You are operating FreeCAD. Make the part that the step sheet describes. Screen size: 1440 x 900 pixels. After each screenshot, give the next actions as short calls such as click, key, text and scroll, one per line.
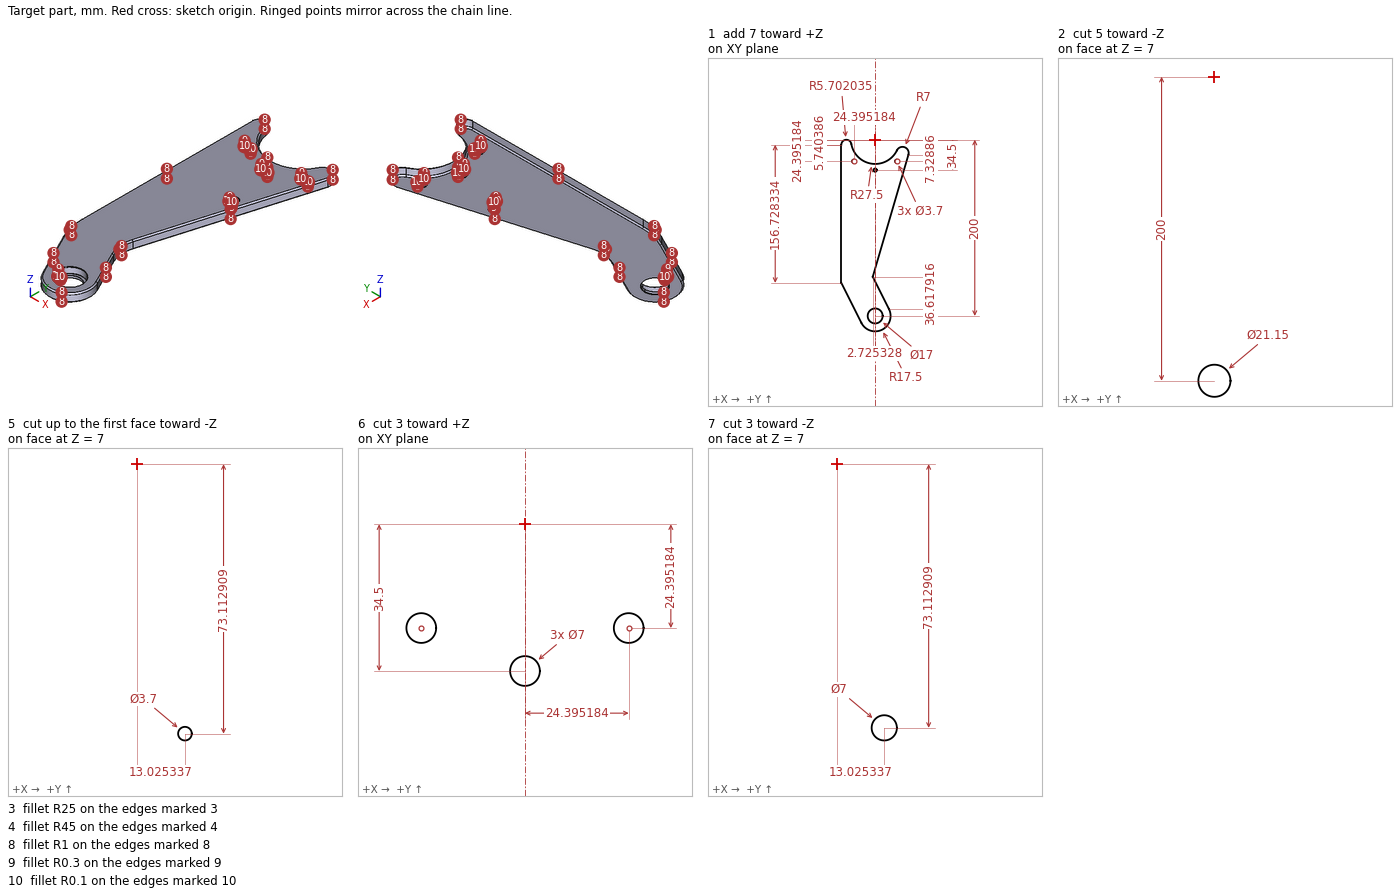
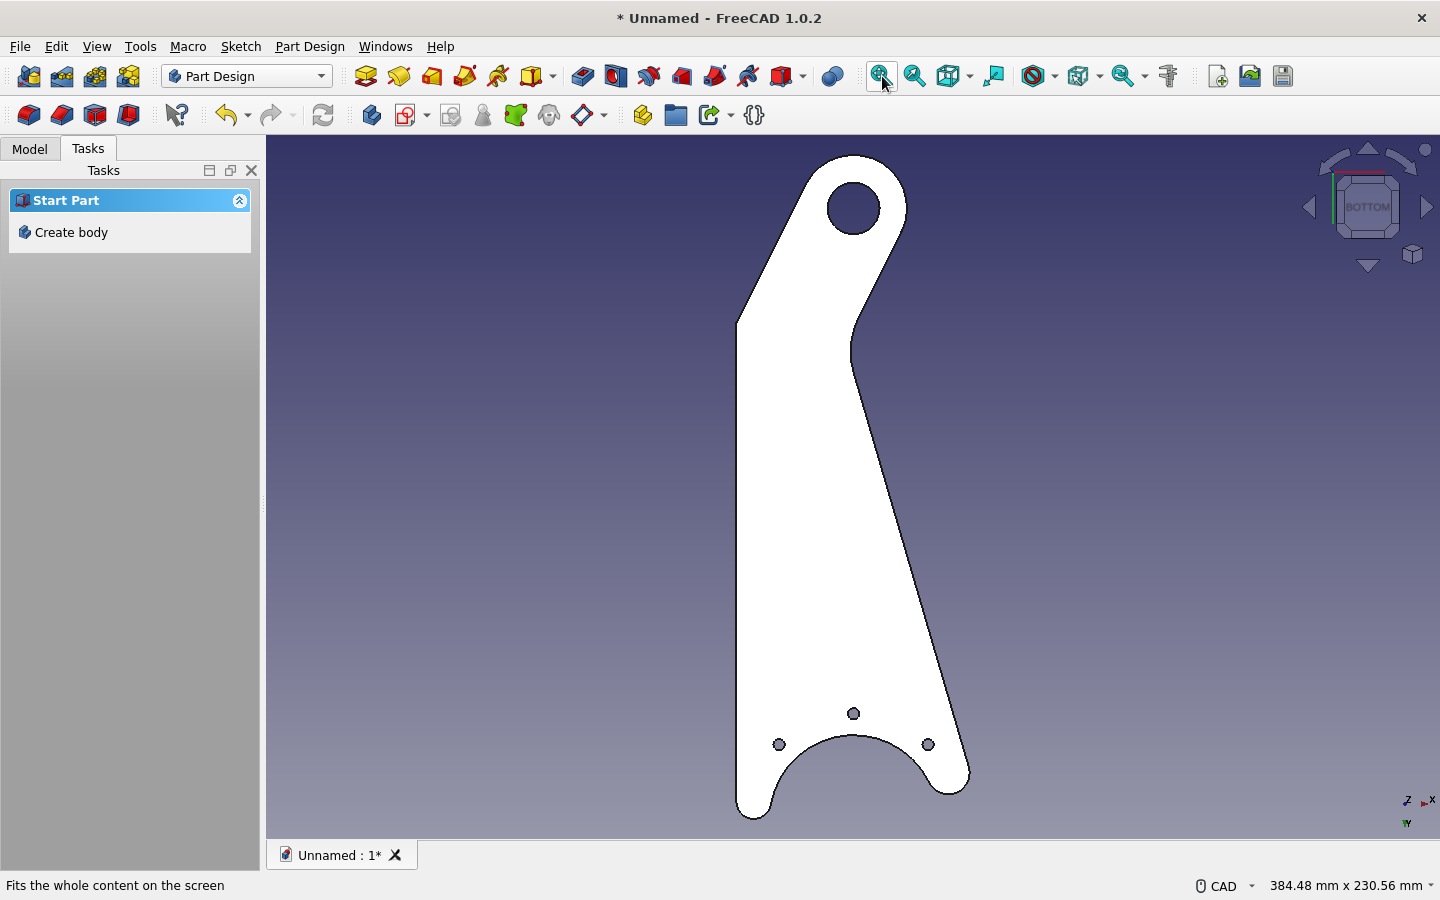
scroll(736, 322, up, 4)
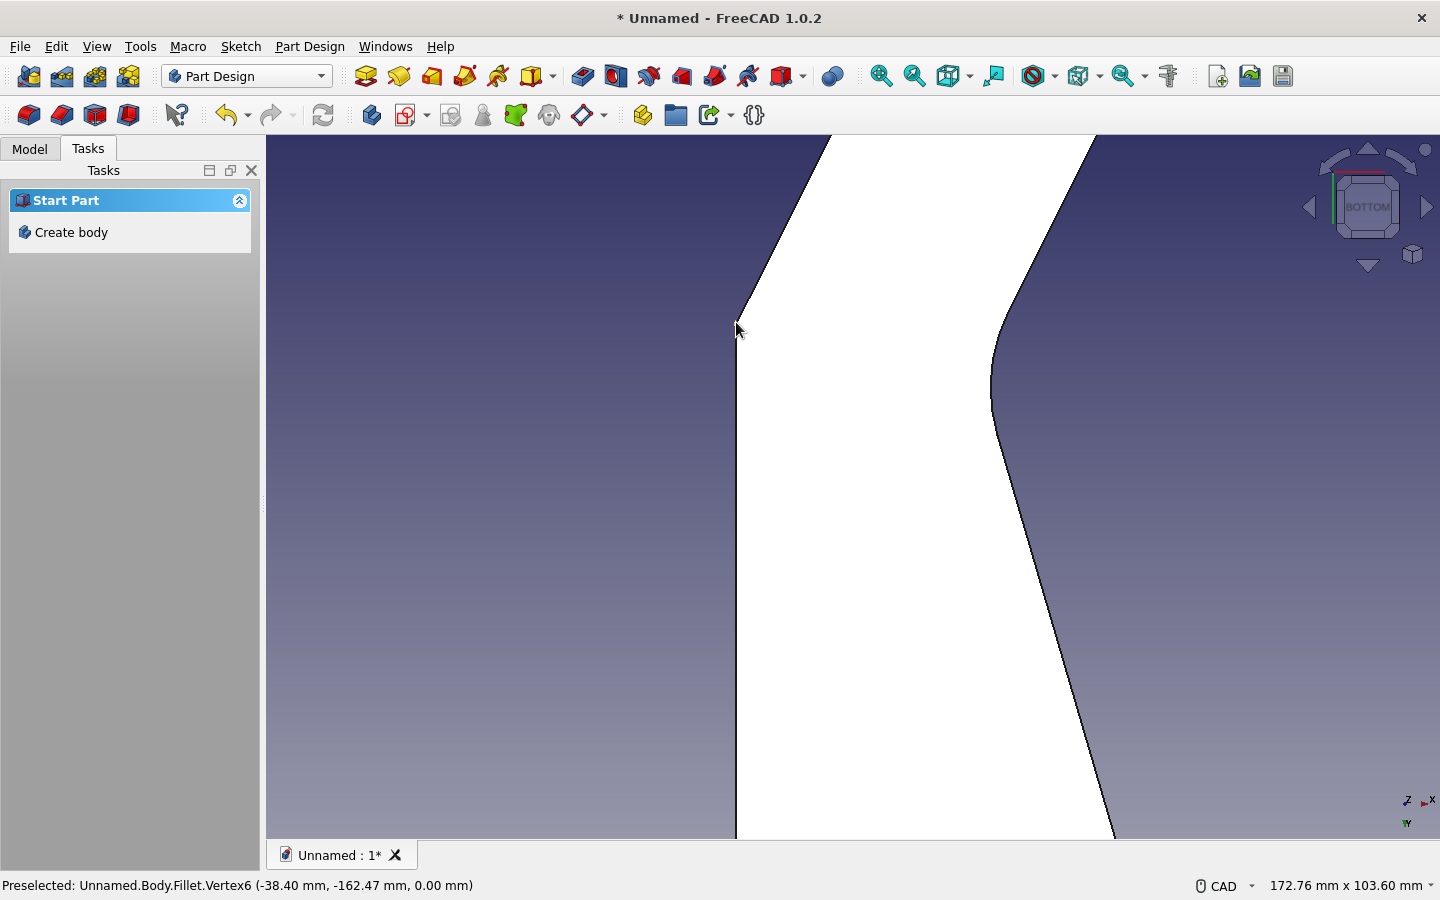
key(v)
key(f)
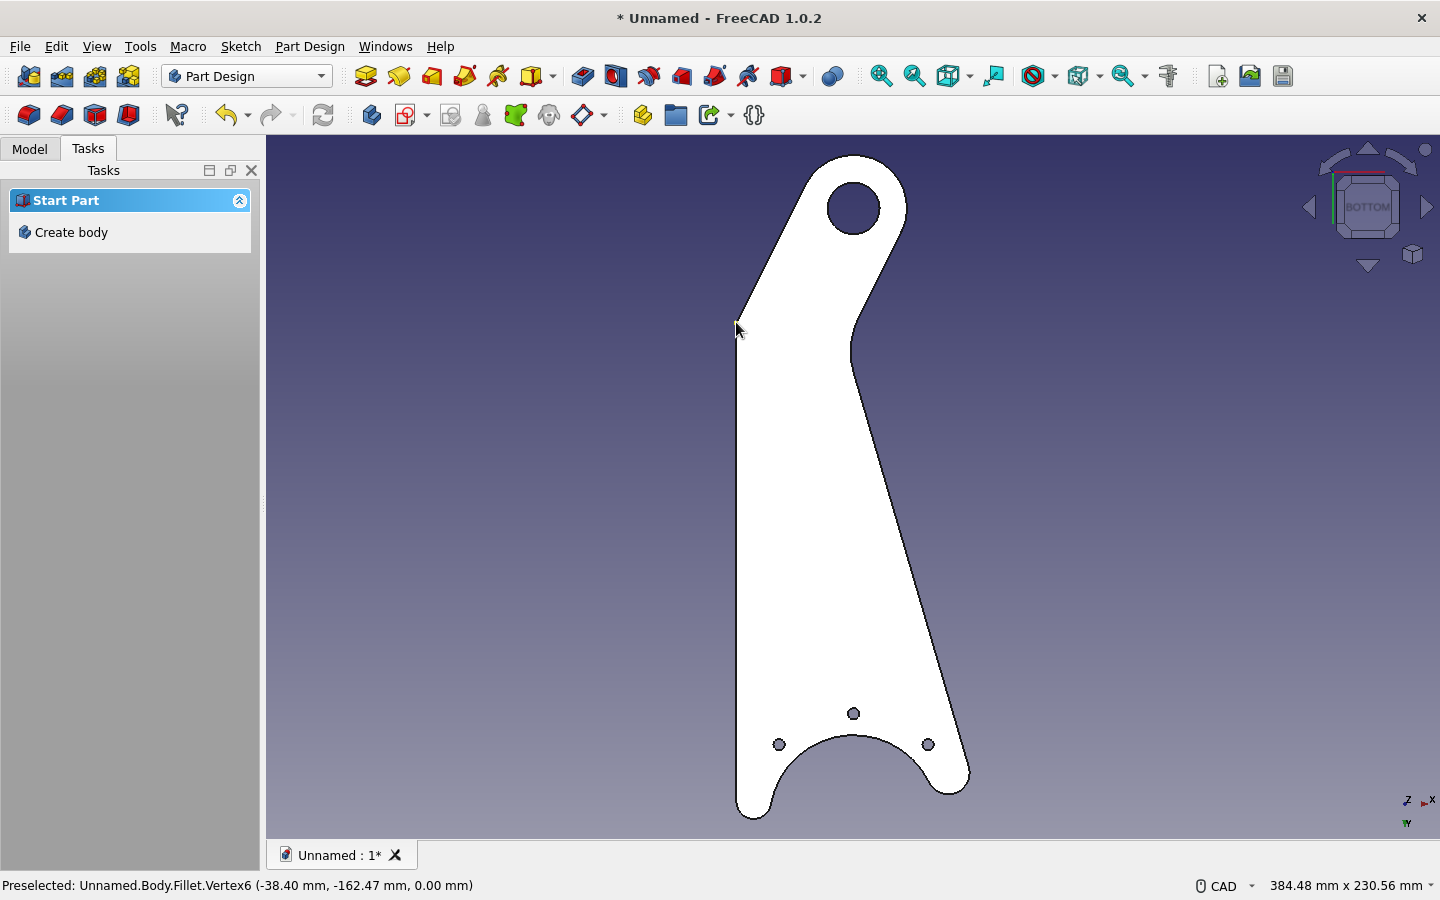
key(4)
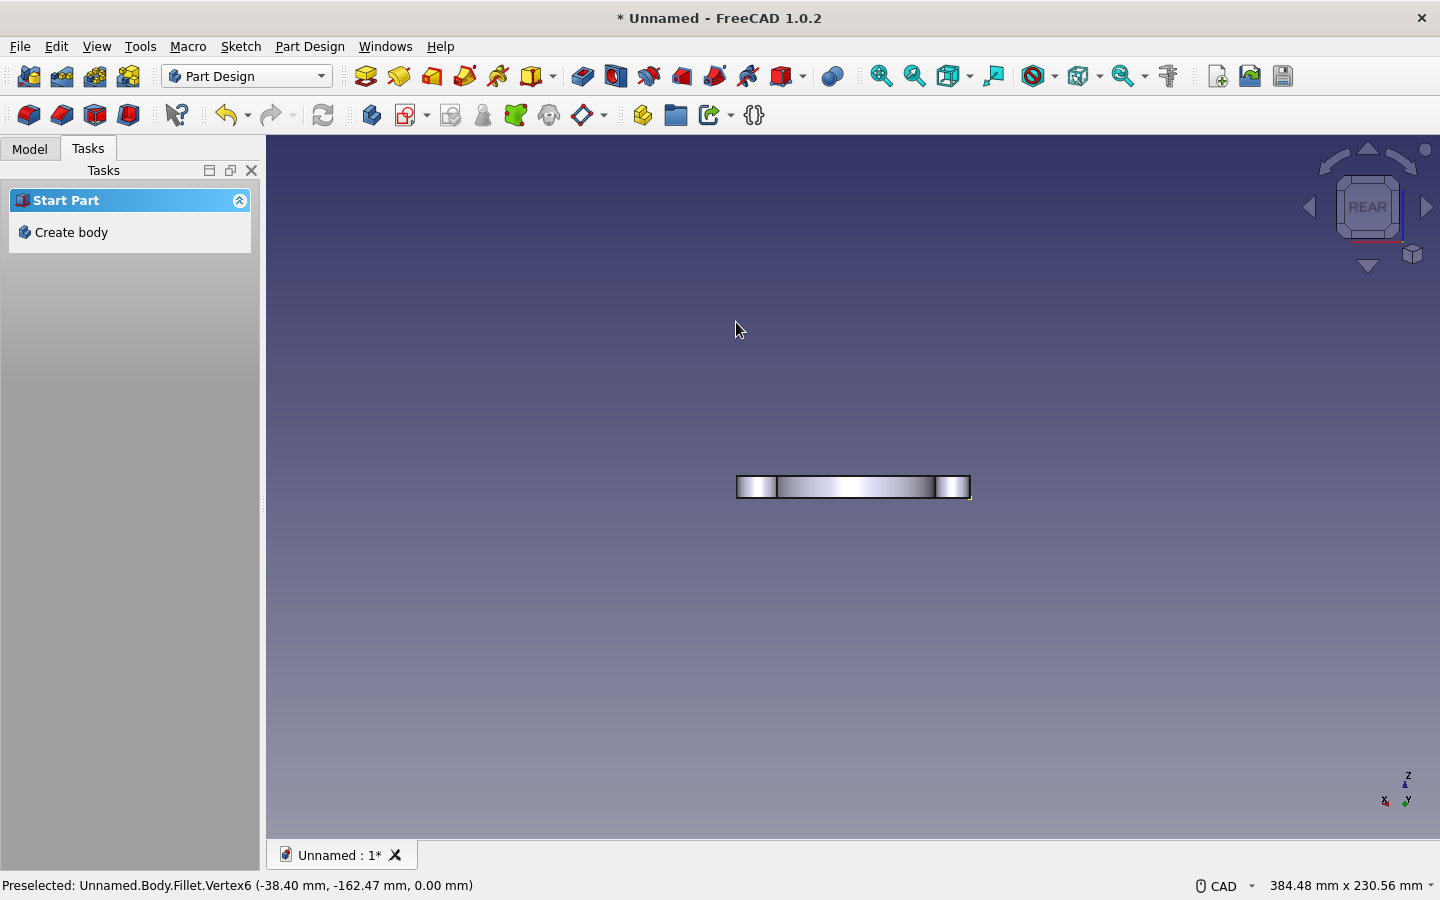
click(882, 76)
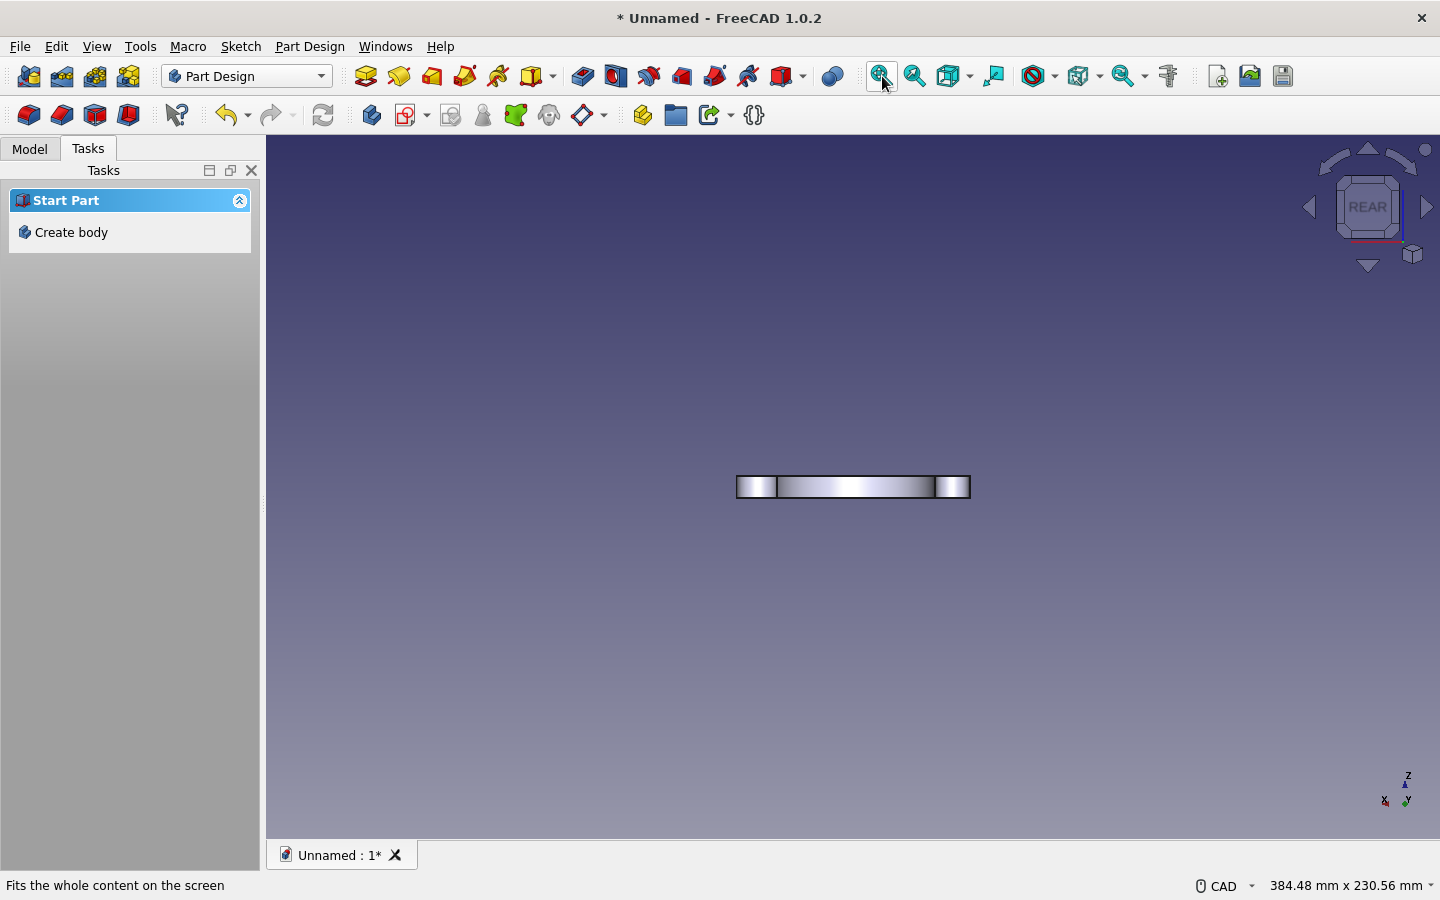
scroll(970, 486, up, 4)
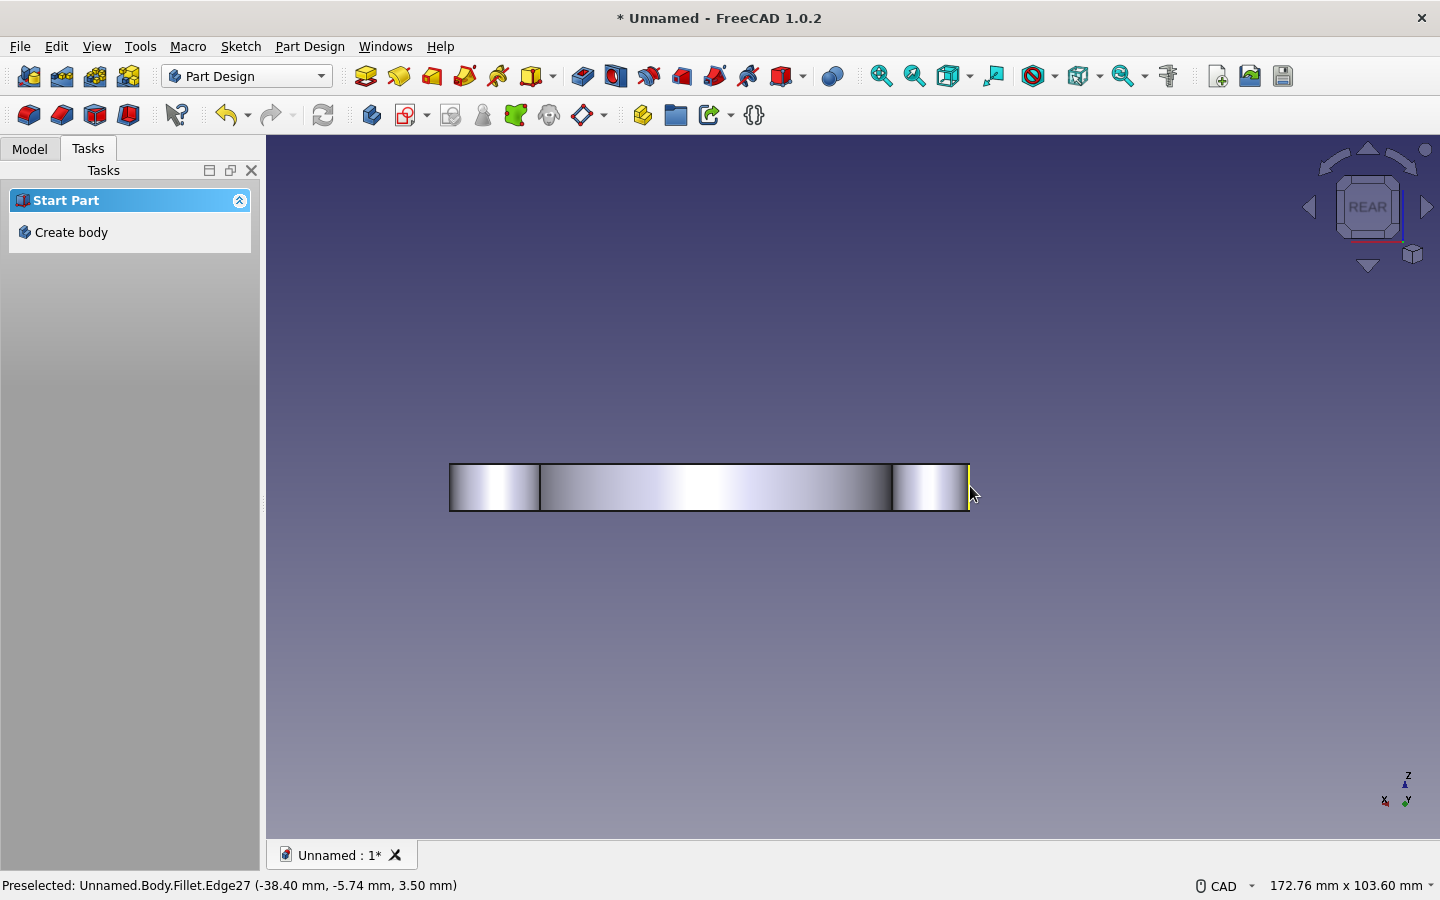
key(v)
key(f)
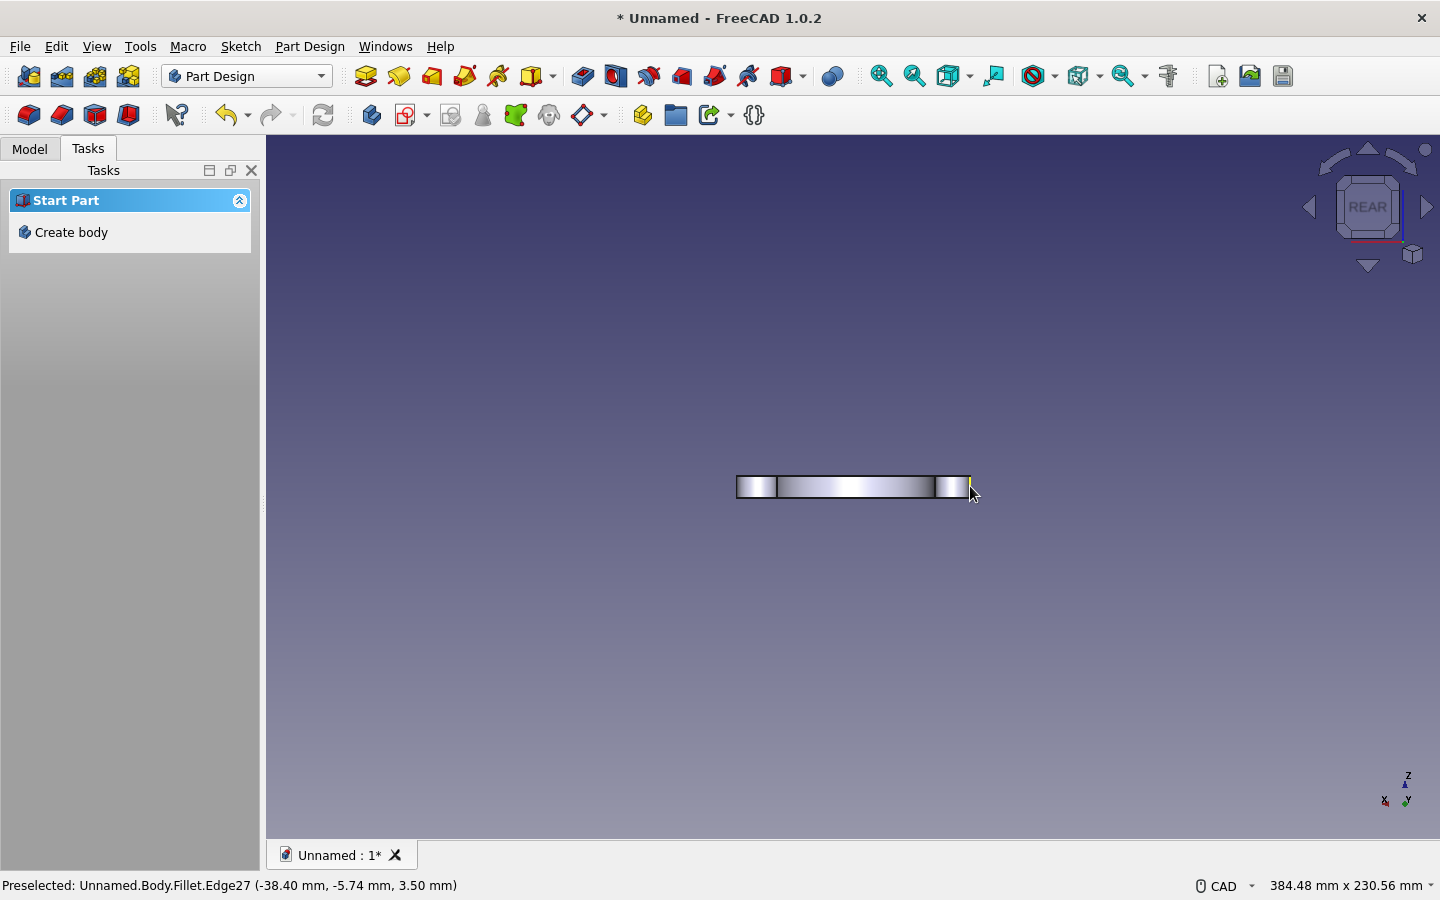
key(6)